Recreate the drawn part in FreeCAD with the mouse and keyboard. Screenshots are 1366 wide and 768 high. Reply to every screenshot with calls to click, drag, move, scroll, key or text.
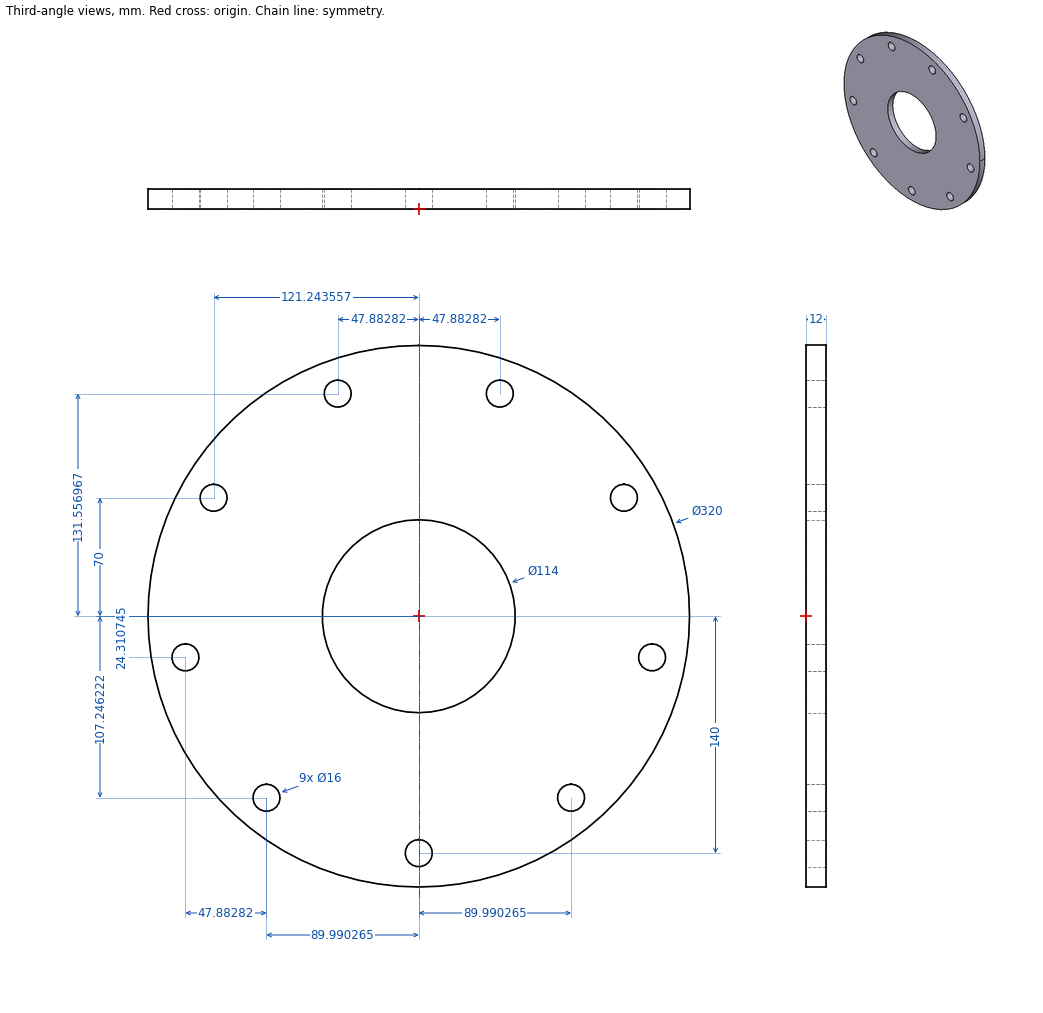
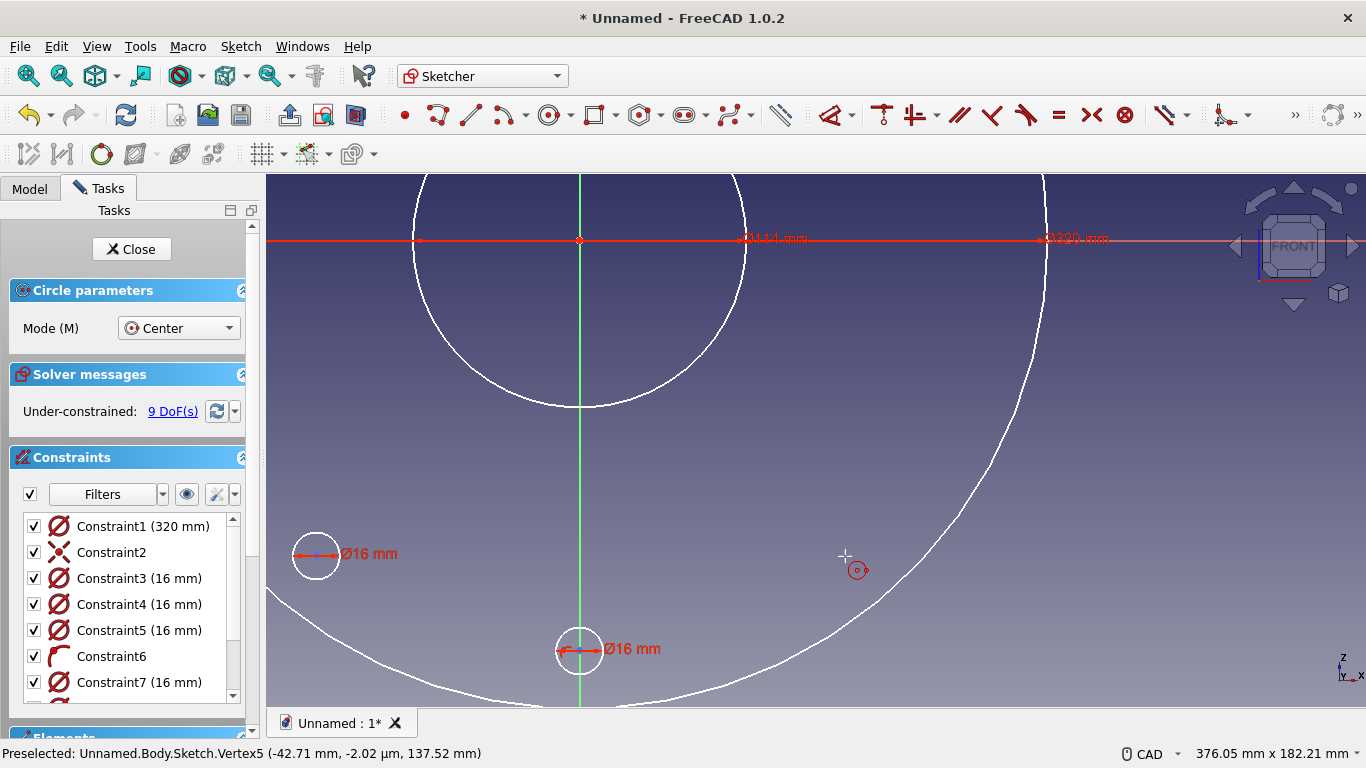
click(843, 555)
move(859, 538)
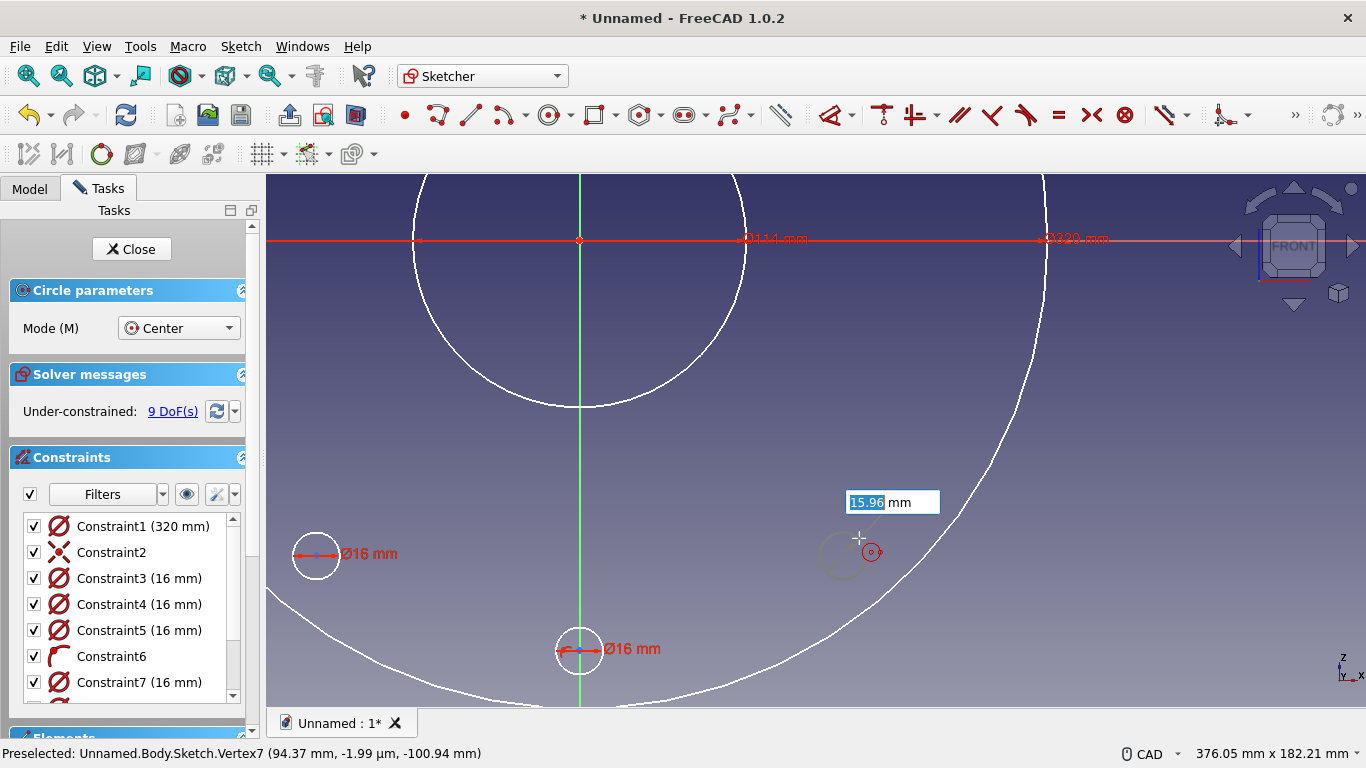
text(16)
key(Return)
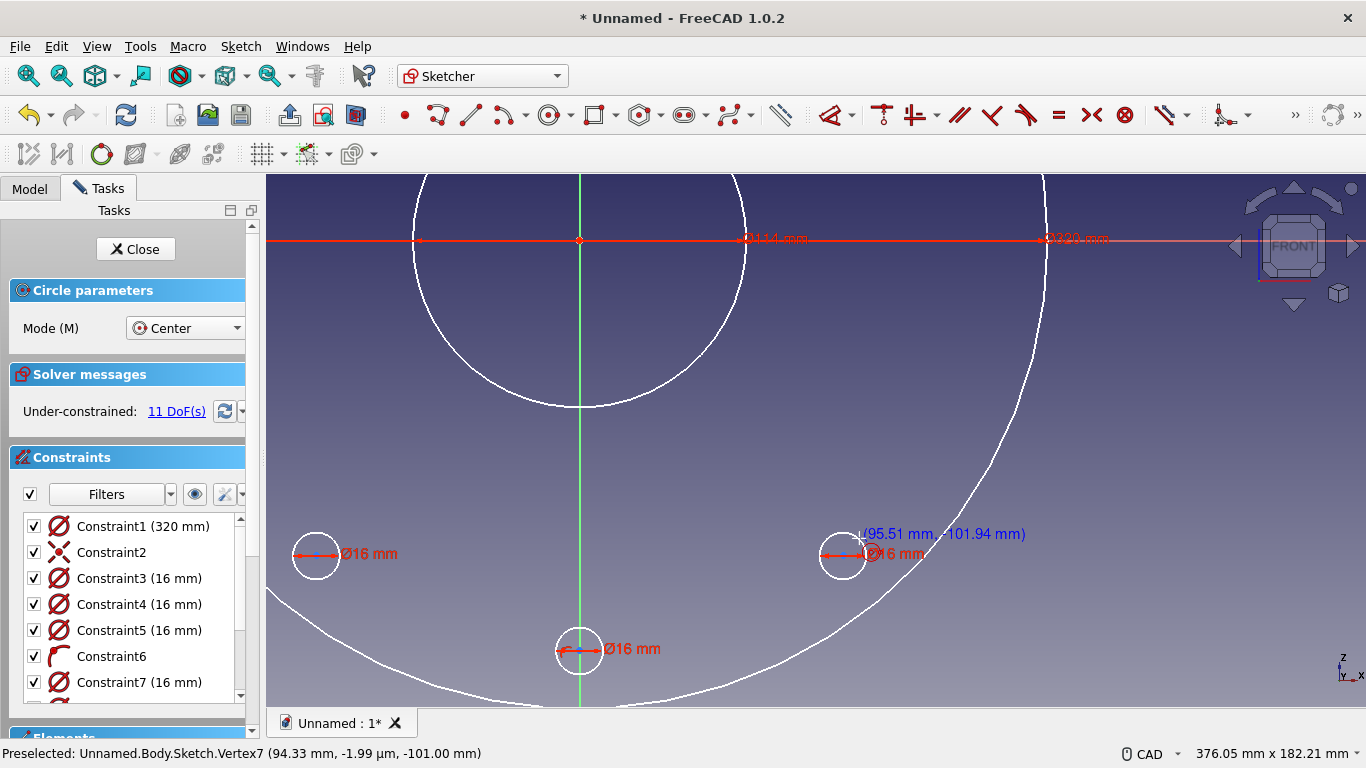
click(983, 312)
move(999, 295)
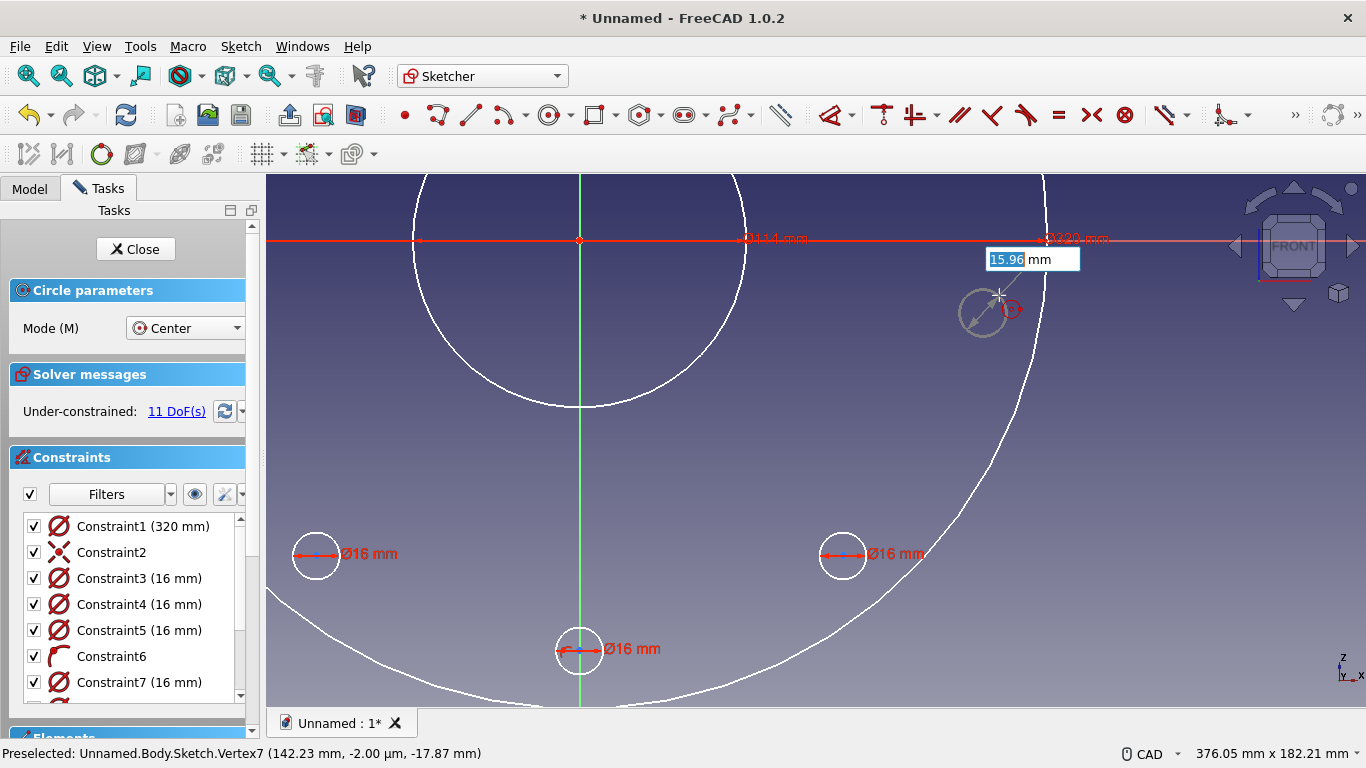
text(16)
key(Return)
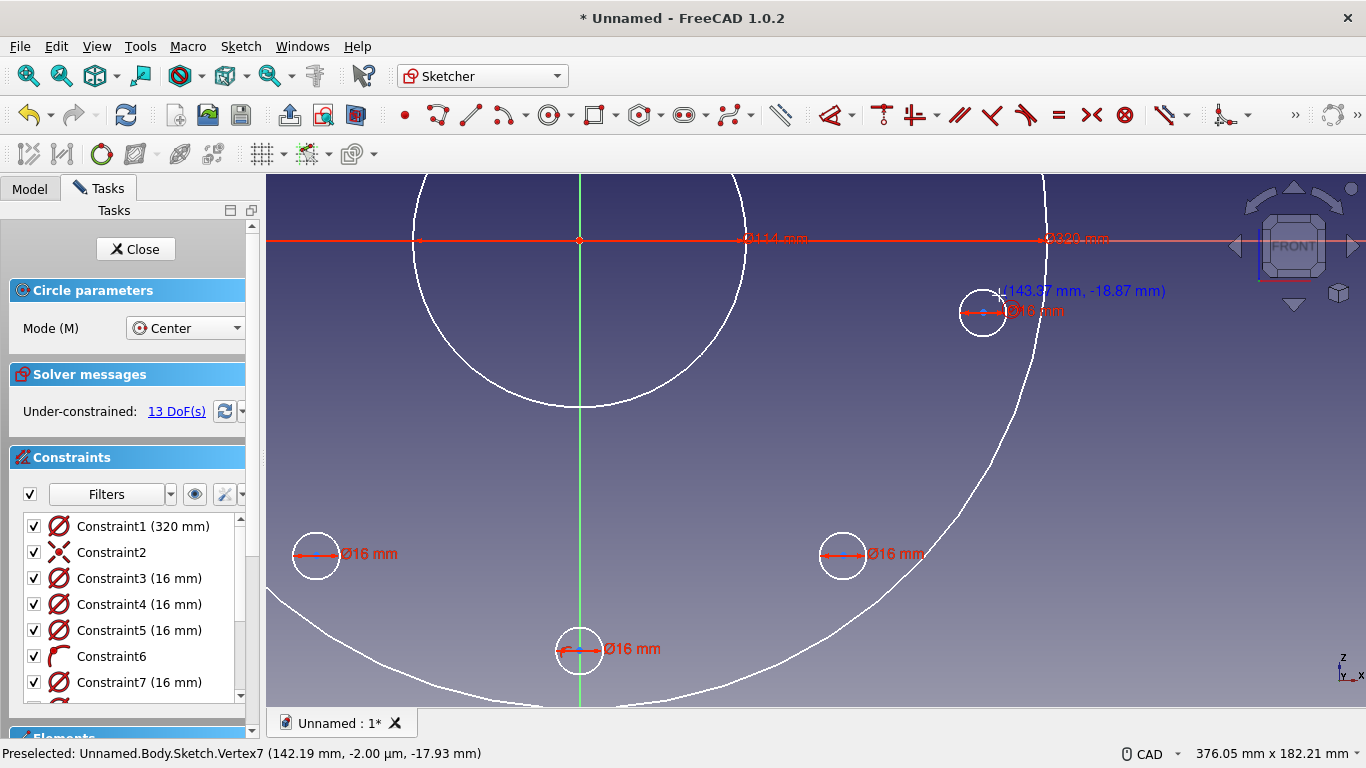
scroll(845, 557, down, 5)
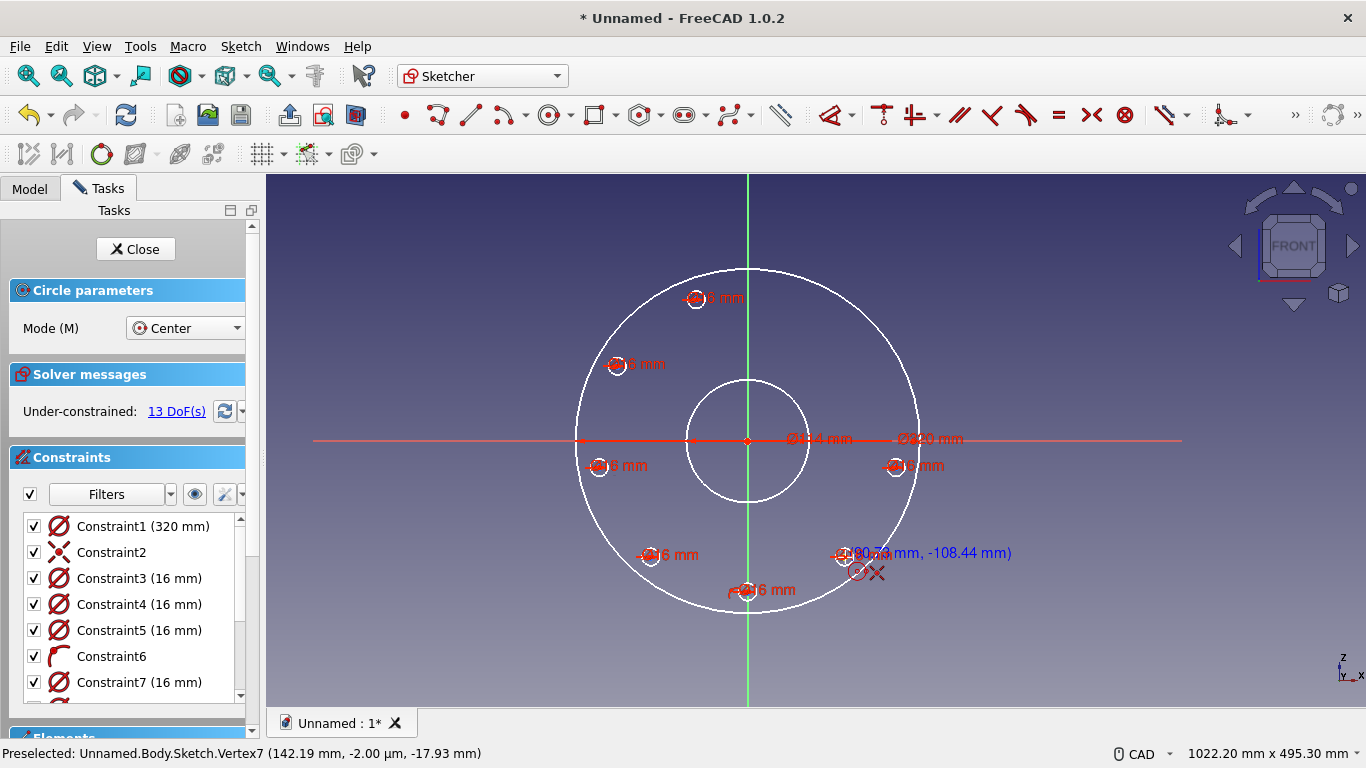
scroll(799, 300, up, 5)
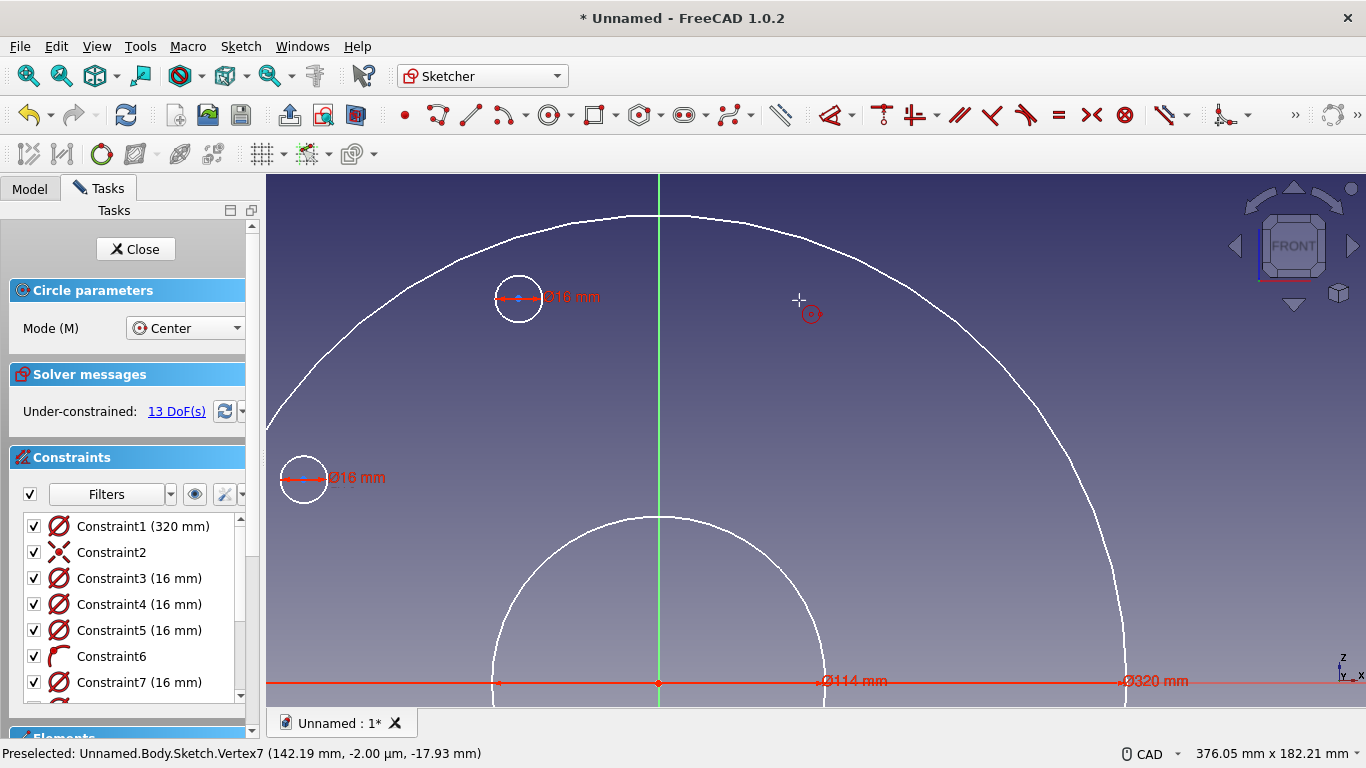
click(799, 298)
move(815, 282)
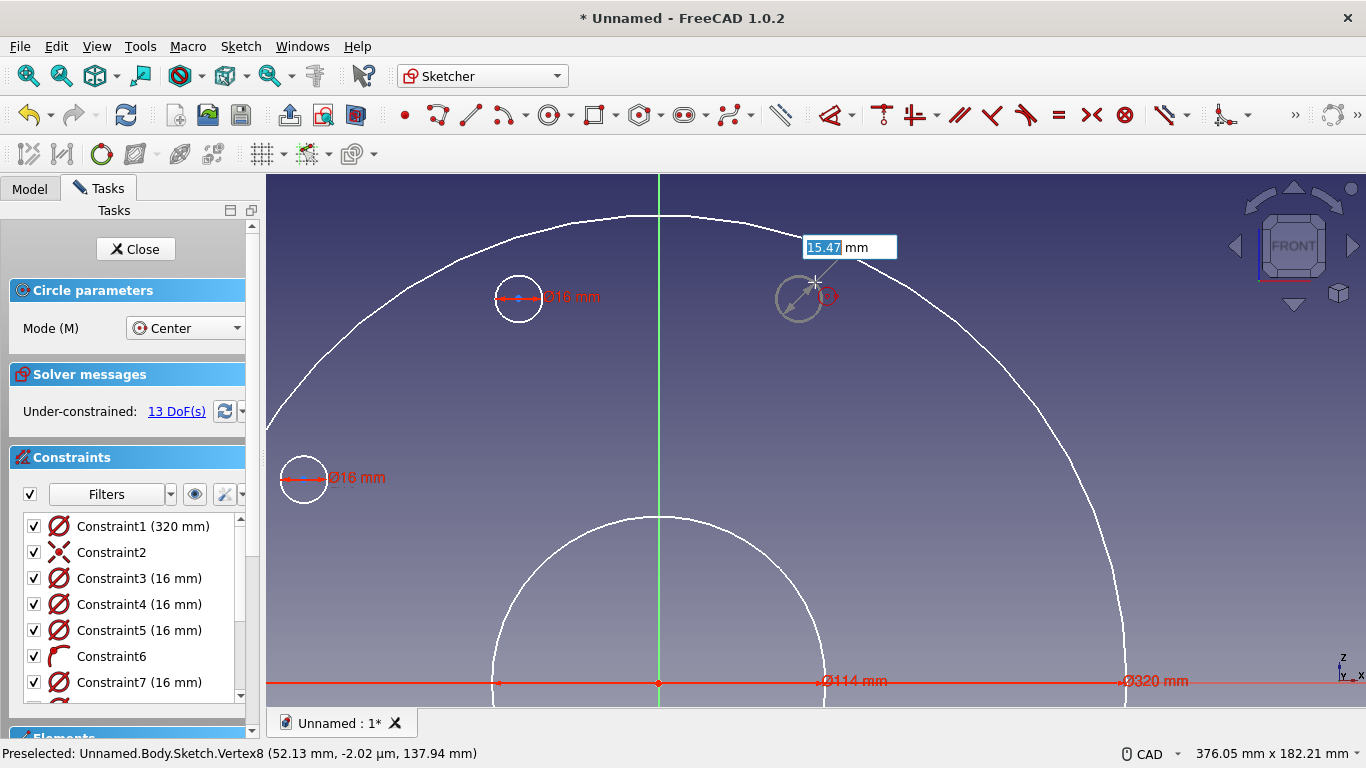
text(16)
key(Return)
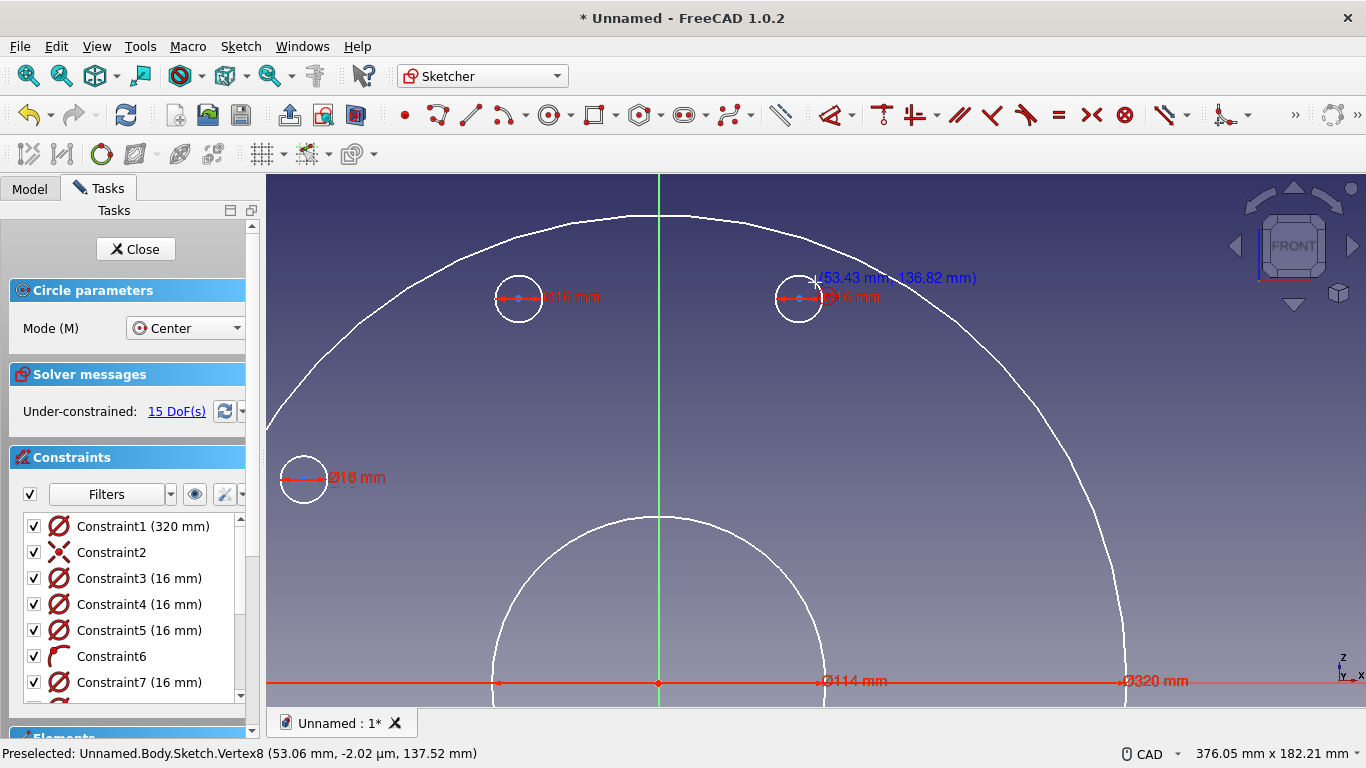
click(1013, 478)
move(1030, 462)